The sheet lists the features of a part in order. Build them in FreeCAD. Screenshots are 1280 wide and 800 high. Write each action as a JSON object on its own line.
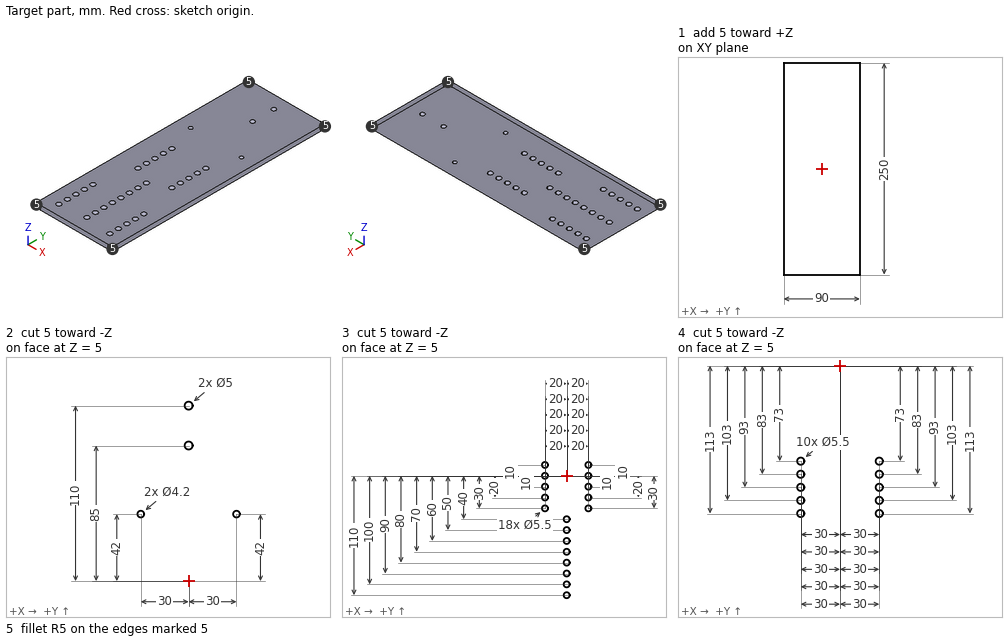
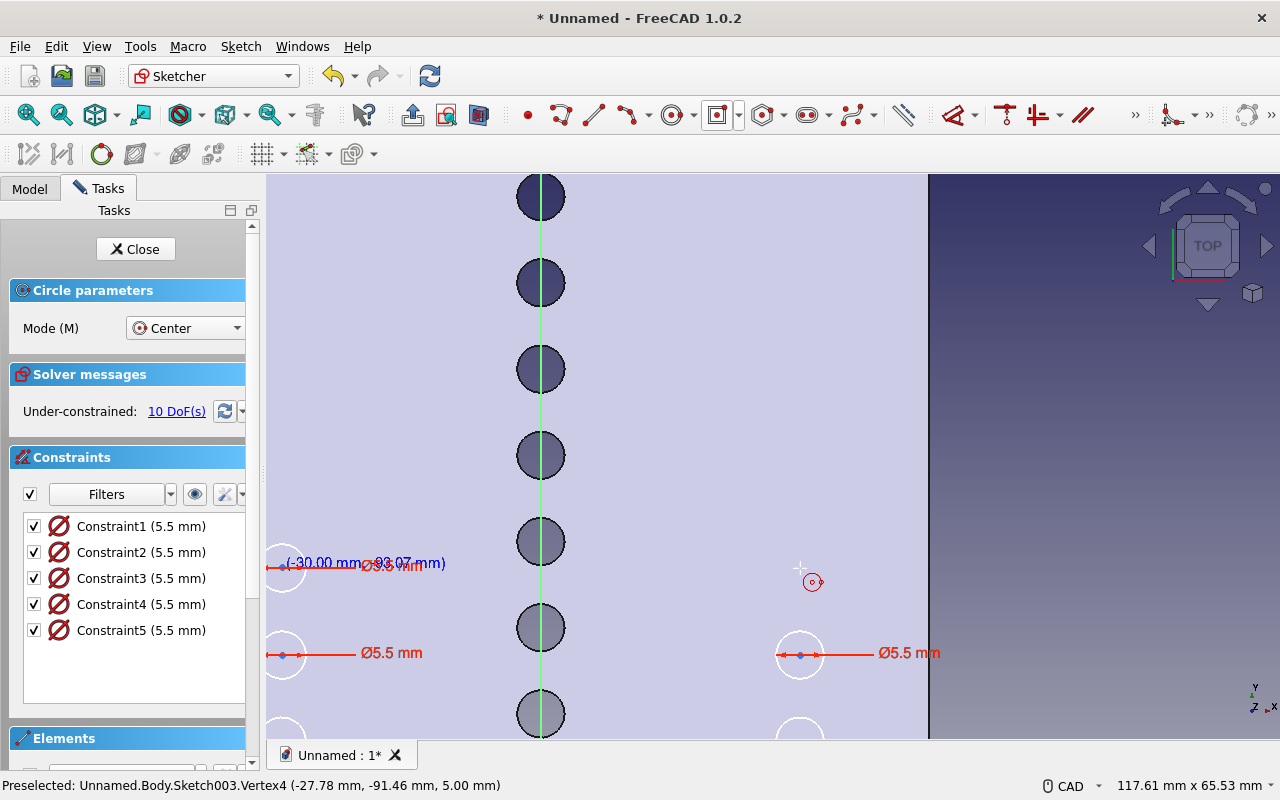
{"action": "left_click", "coordinate": [800, 567]}
{"action": "mouse_move", "coordinate": [816, 551]}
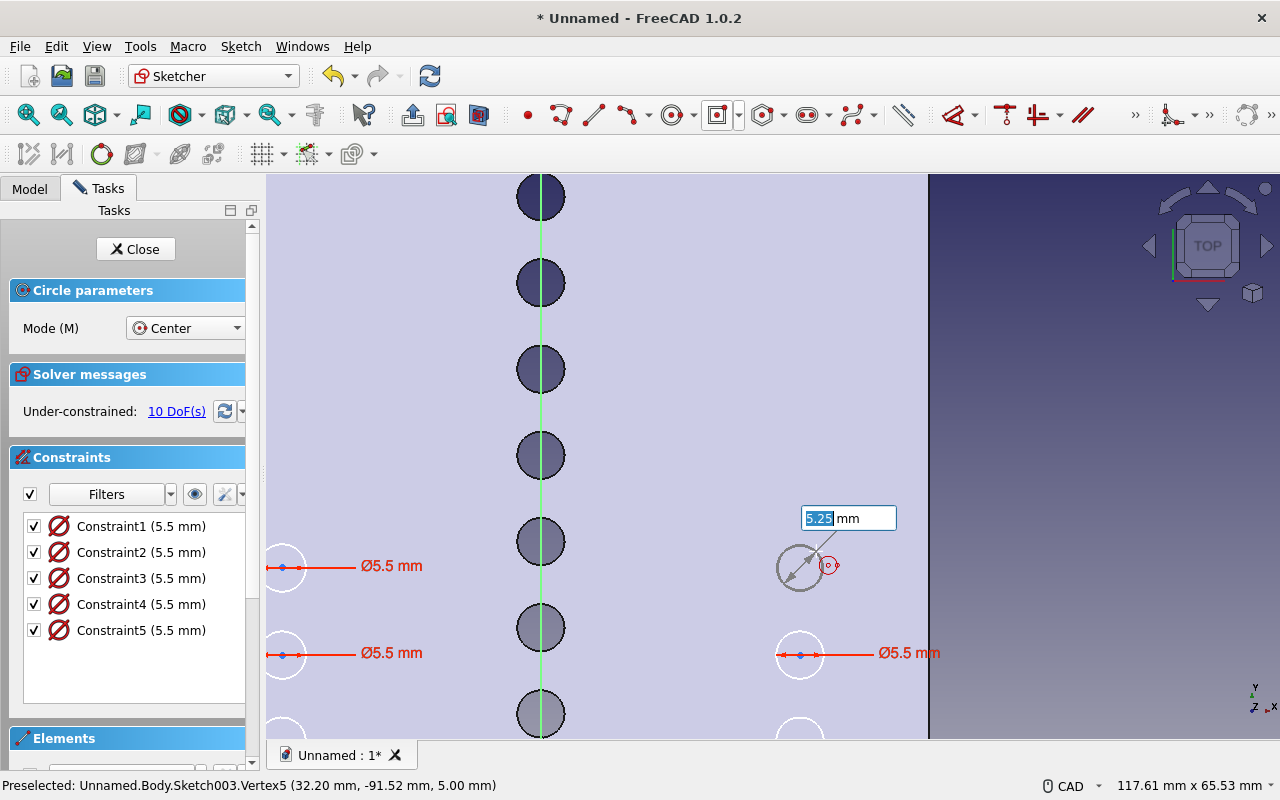
{"action": "type", "text": "5.5"}
{"action": "key", "text": "Return"}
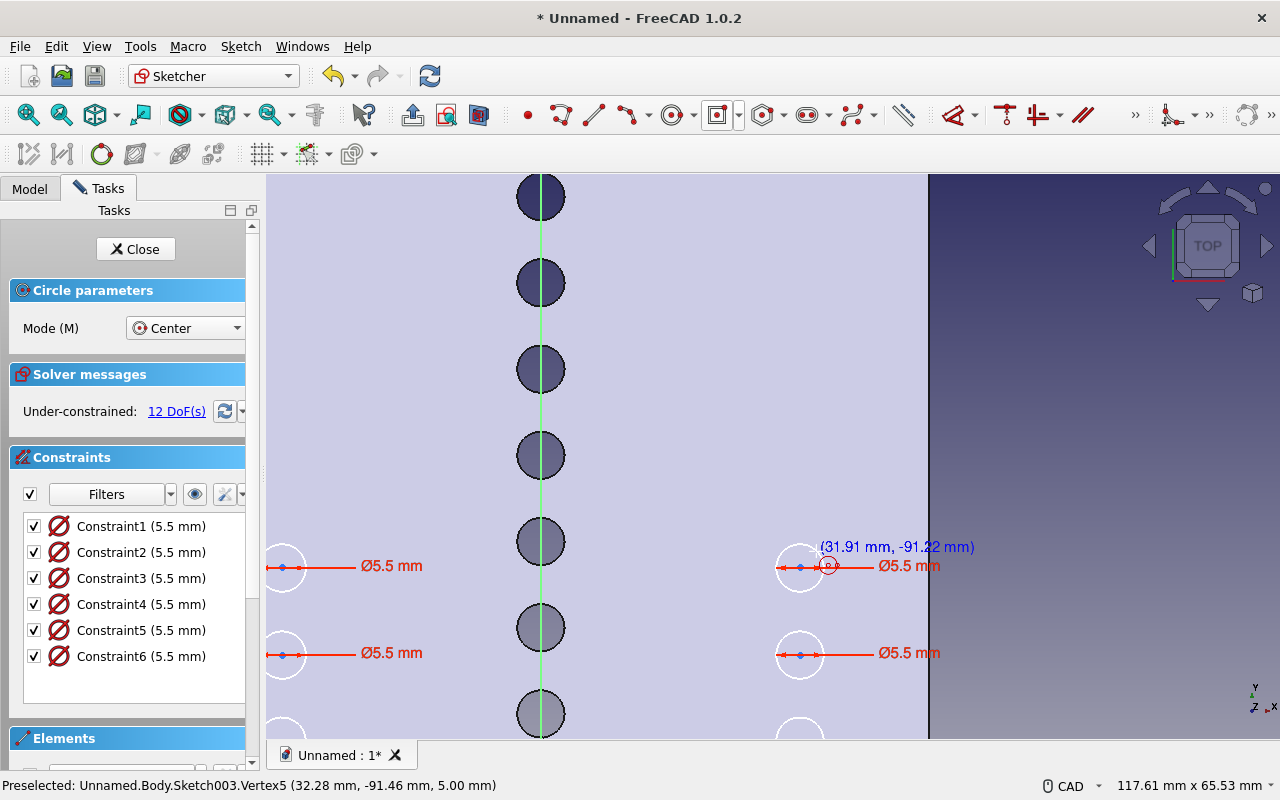
{"action": "scroll", "coordinate": [800, 568], "scroll_direction": "down", "scroll_amount": 5}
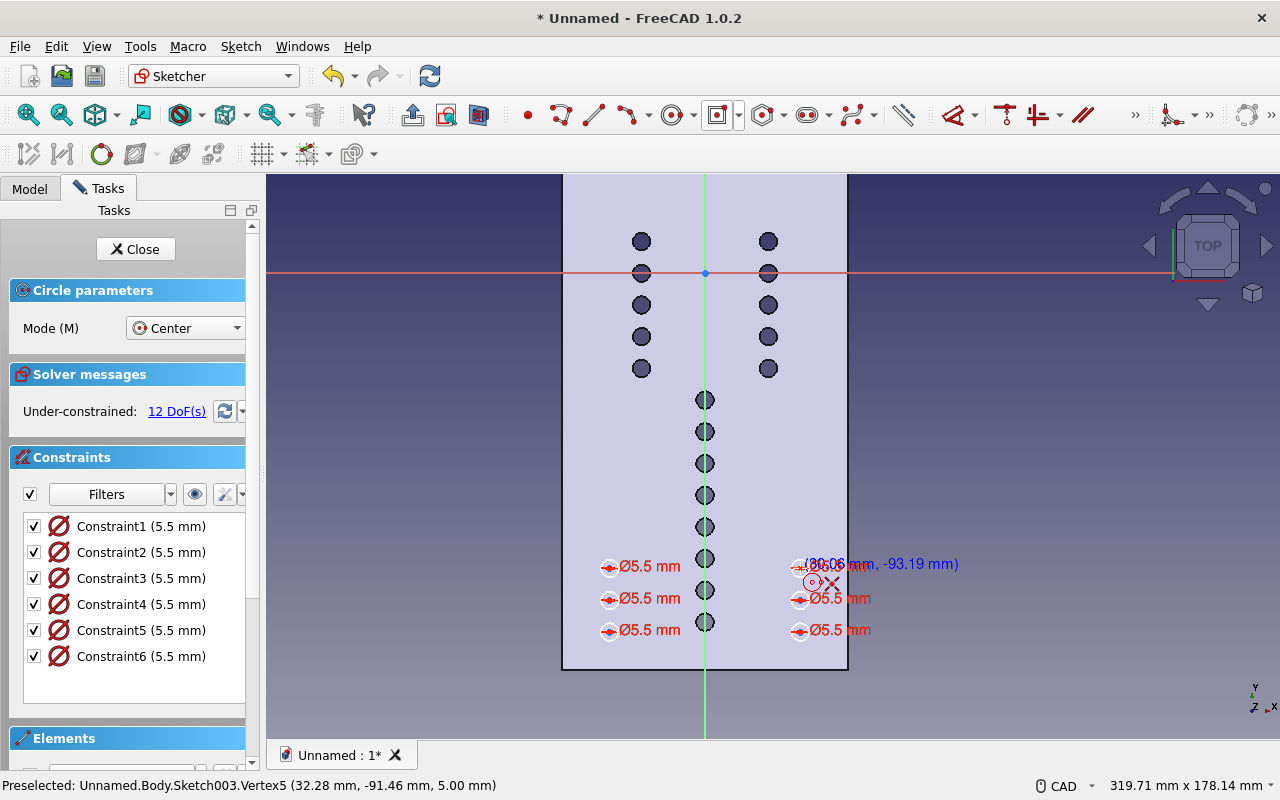
{"action": "scroll", "coordinate": [610, 536], "scroll_direction": "up", "scroll_amount": 5}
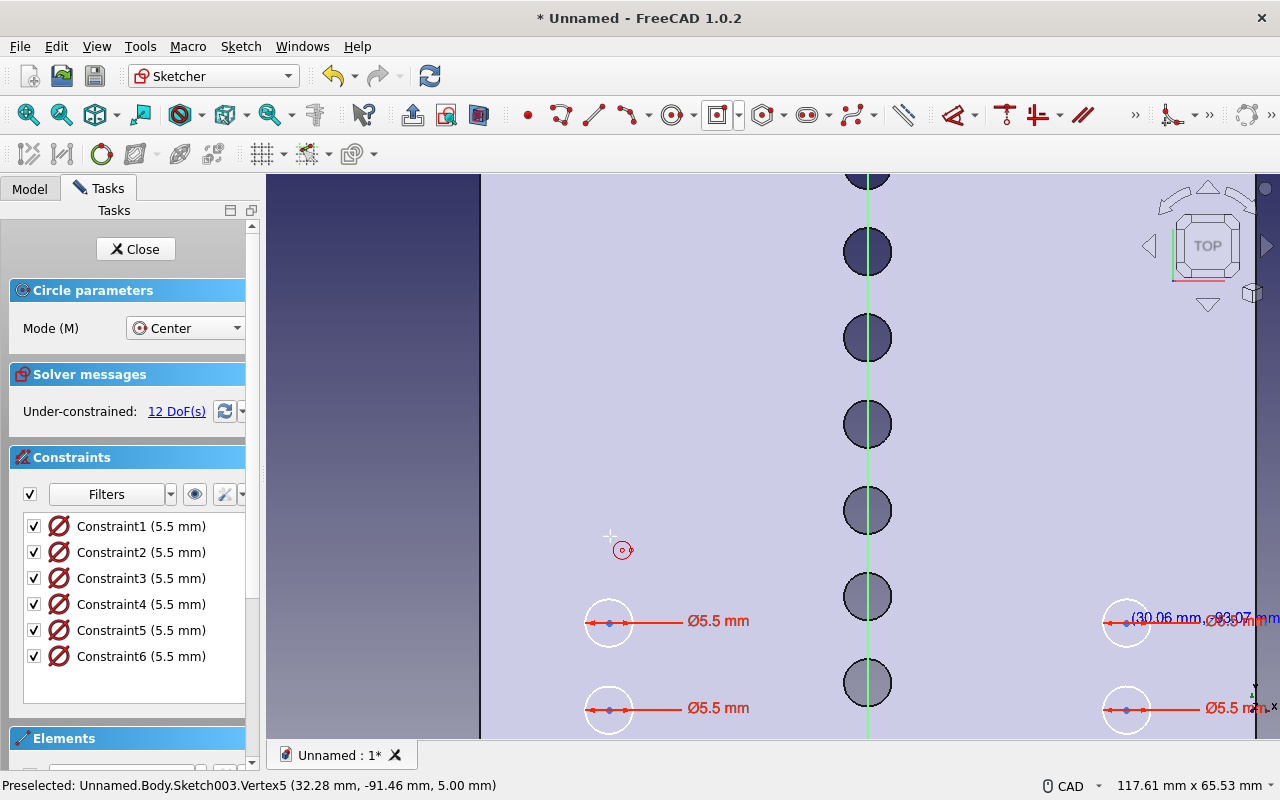
{"action": "left_click", "coordinate": [609, 536]}
{"action": "mouse_move", "coordinate": [626, 519]}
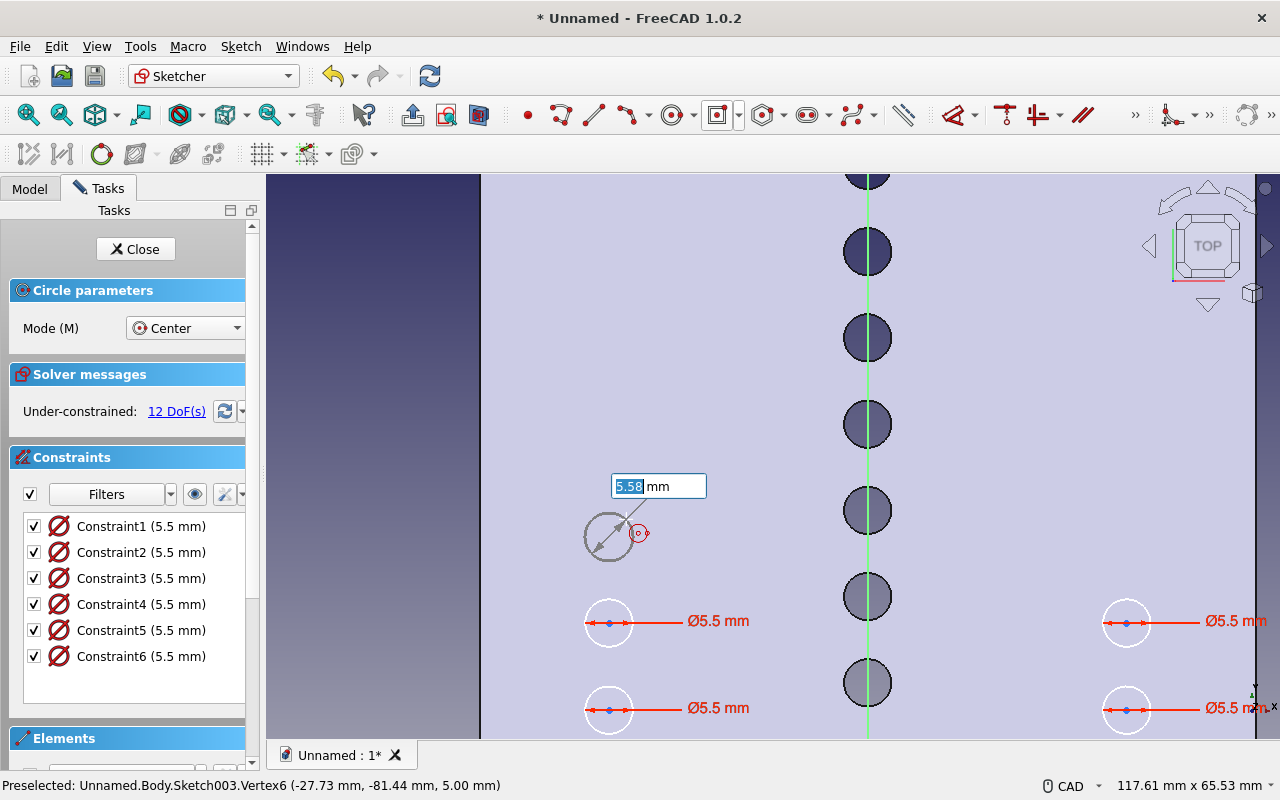
{"action": "type", "text": "5.5"}
{"action": "key", "text": "Return"}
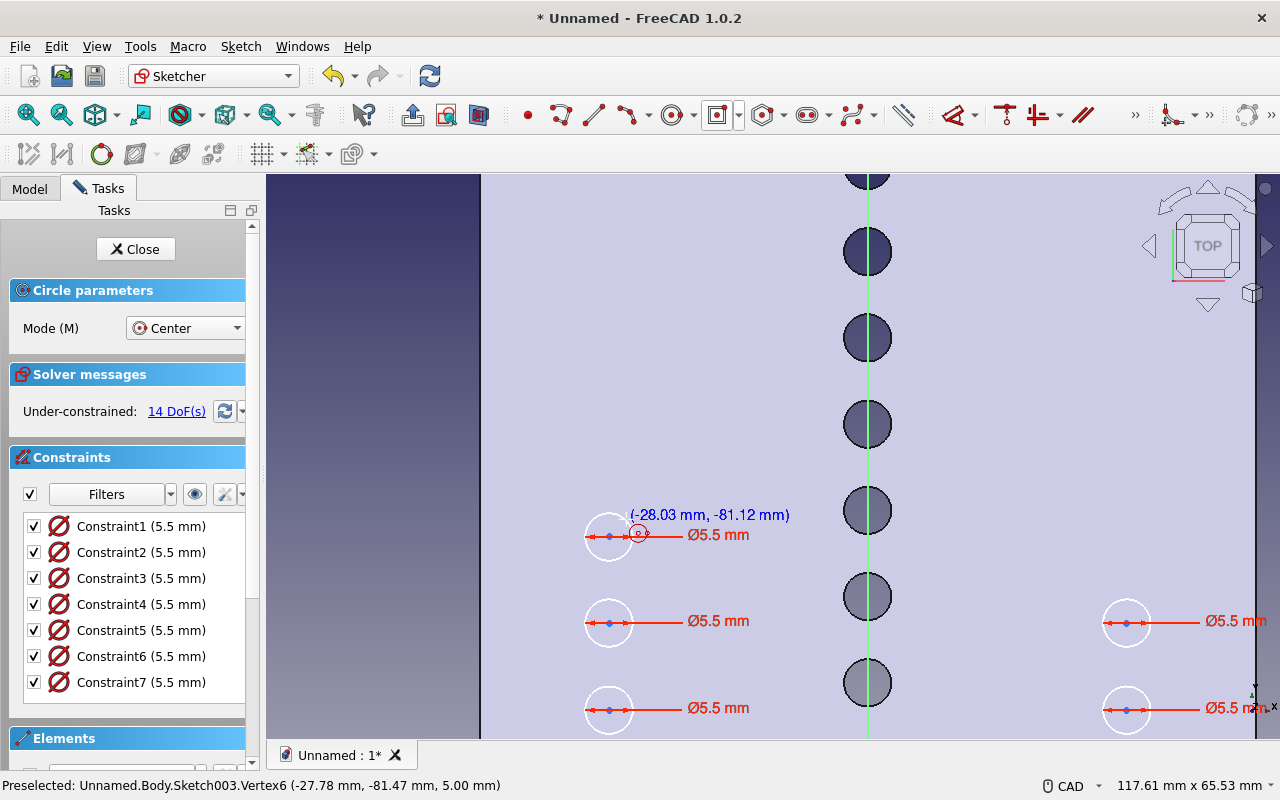
{"action": "scroll", "coordinate": [610, 536], "scroll_direction": "down", "scroll_amount": 5}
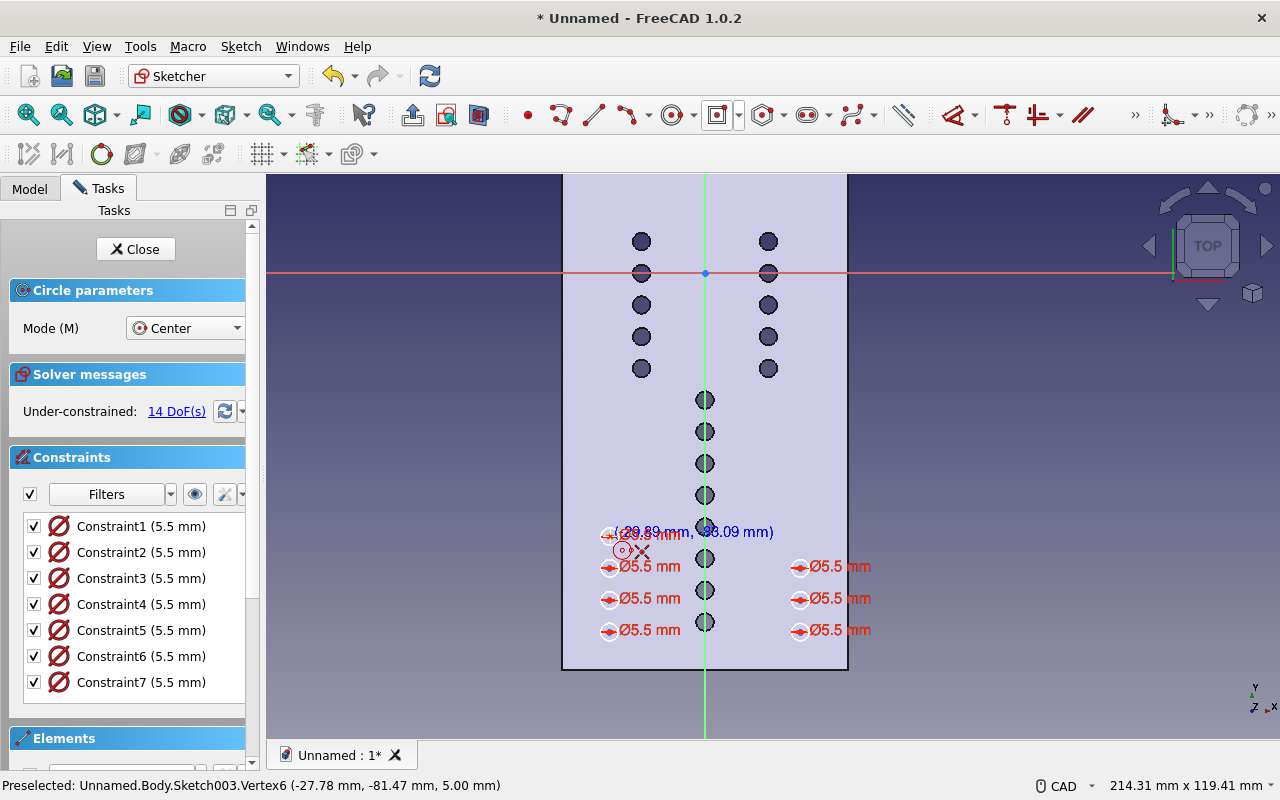
{"action": "scroll", "coordinate": [800, 536], "scroll_direction": "up", "scroll_amount": 5}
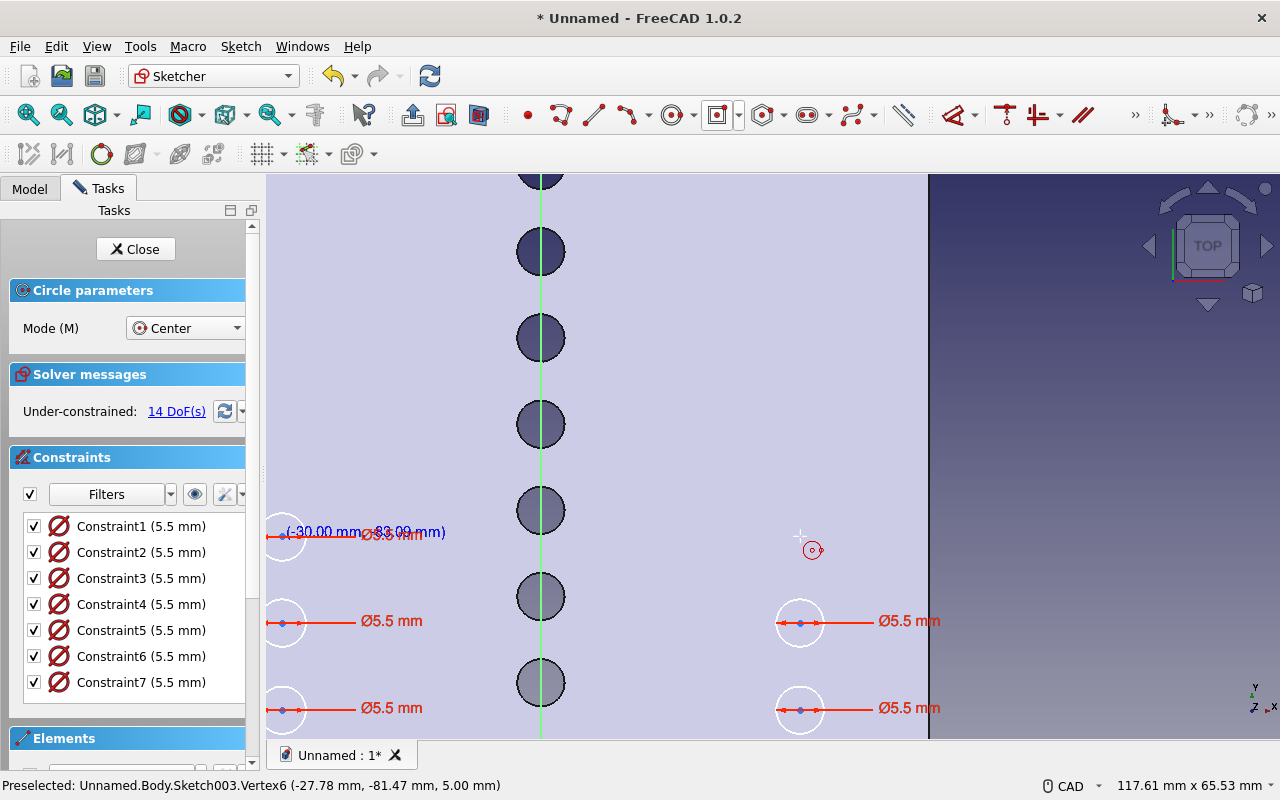
{"action": "left_click", "coordinate": [800, 536]}
{"action": "mouse_move", "coordinate": [816, 519]}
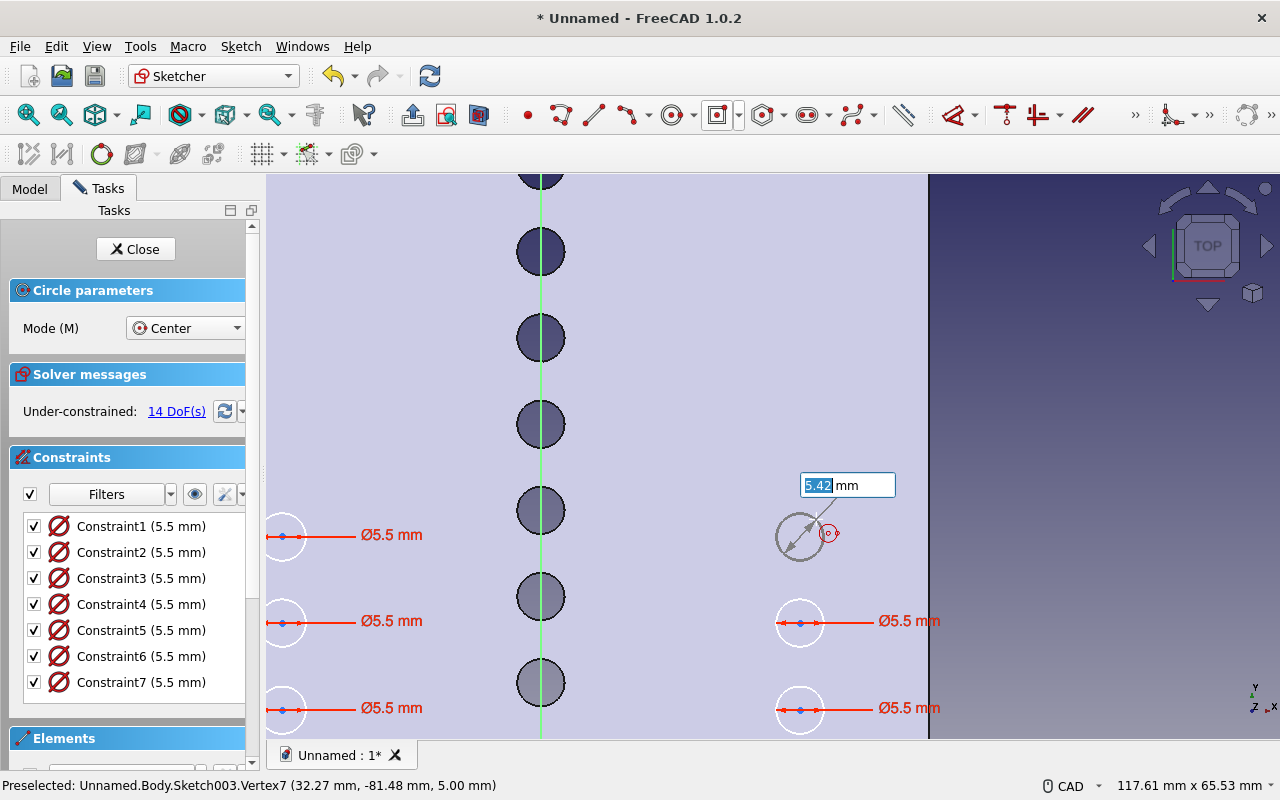
{"action": "type", "text": "5.5"}
{"action": "key", "text": "Return"}